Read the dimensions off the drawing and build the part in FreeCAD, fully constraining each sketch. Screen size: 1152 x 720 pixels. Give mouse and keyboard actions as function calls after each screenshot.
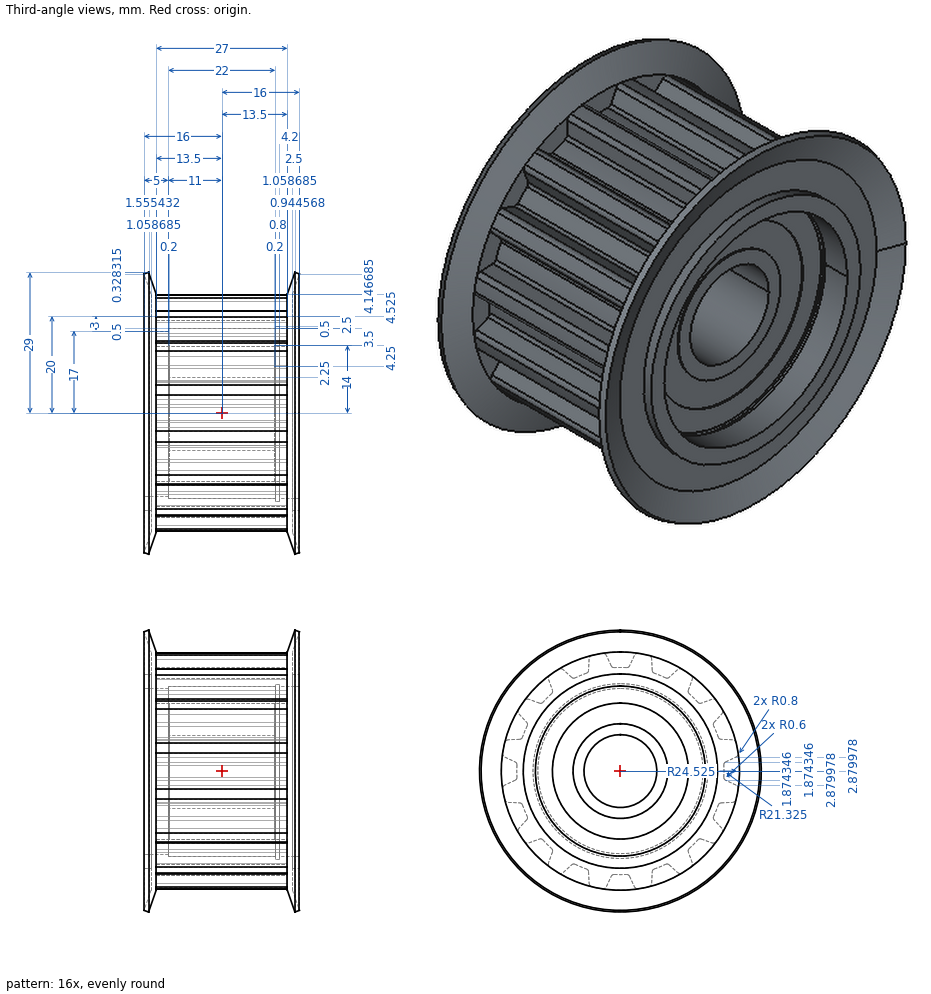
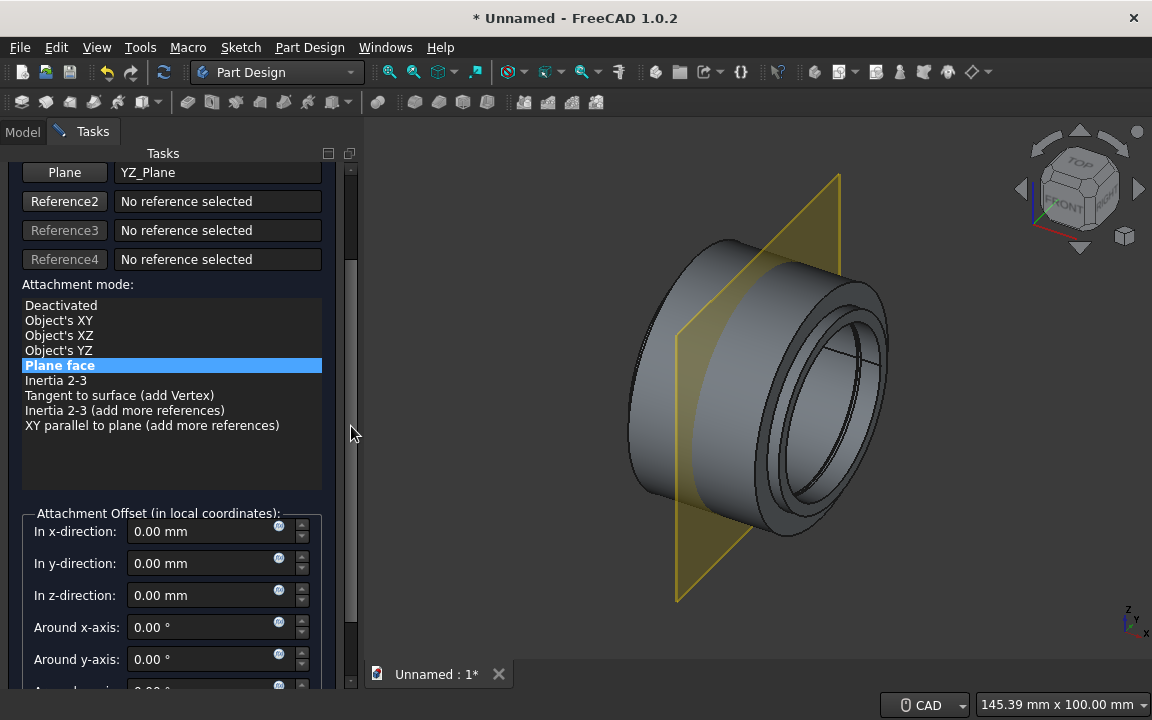
triple_click(210, 595)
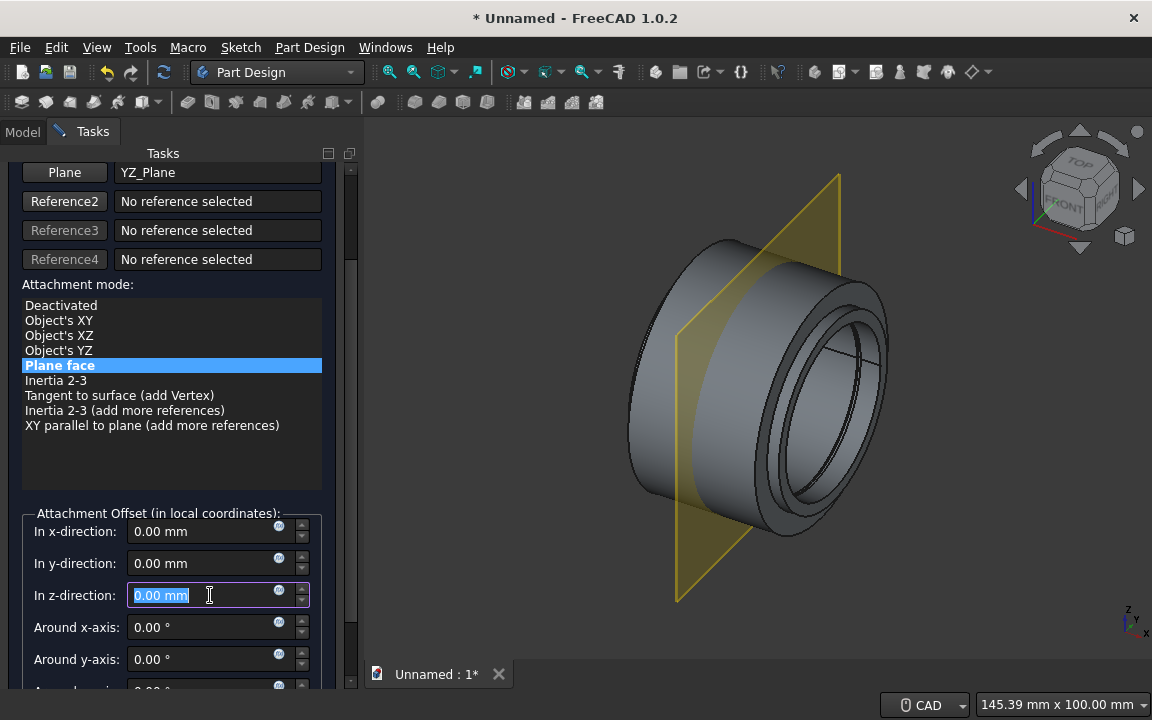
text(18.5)
key(Tab)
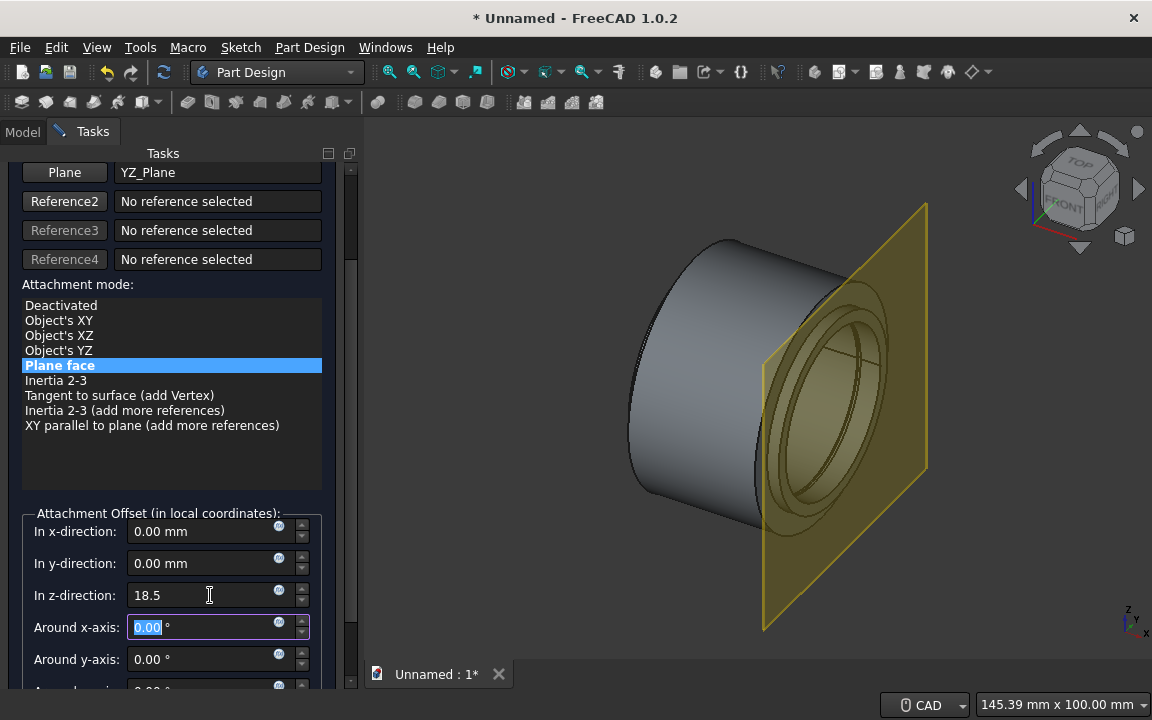
scroll(351, 426, up, 3)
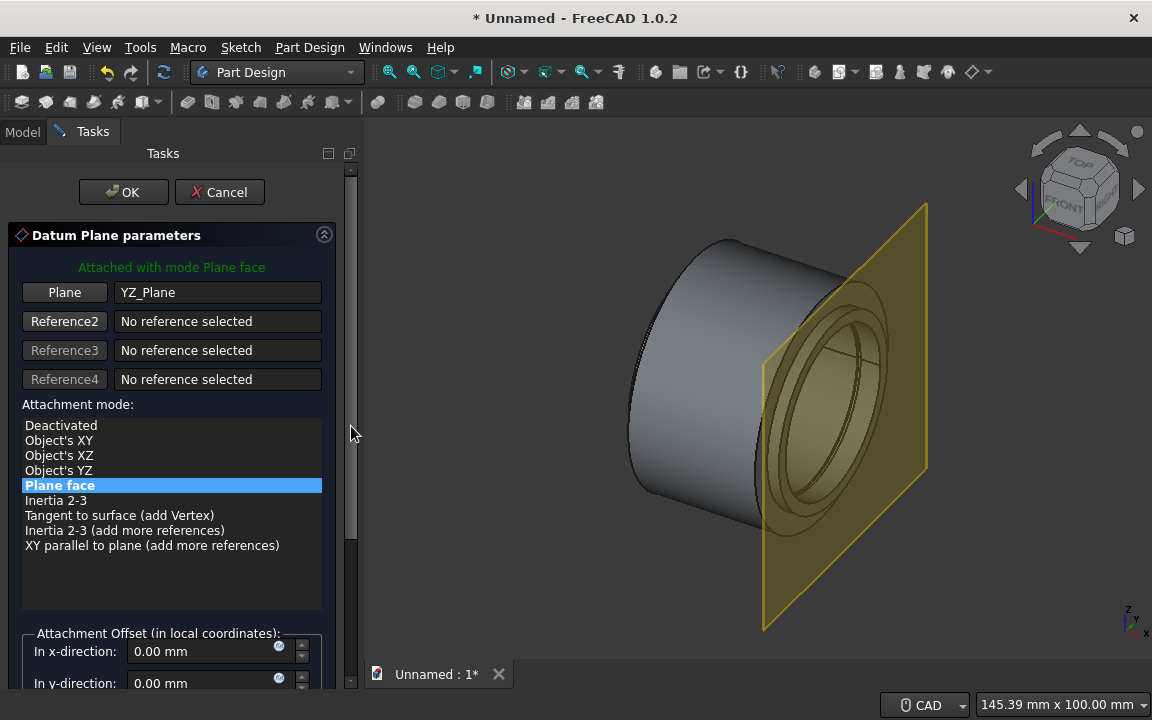
click(124, 192)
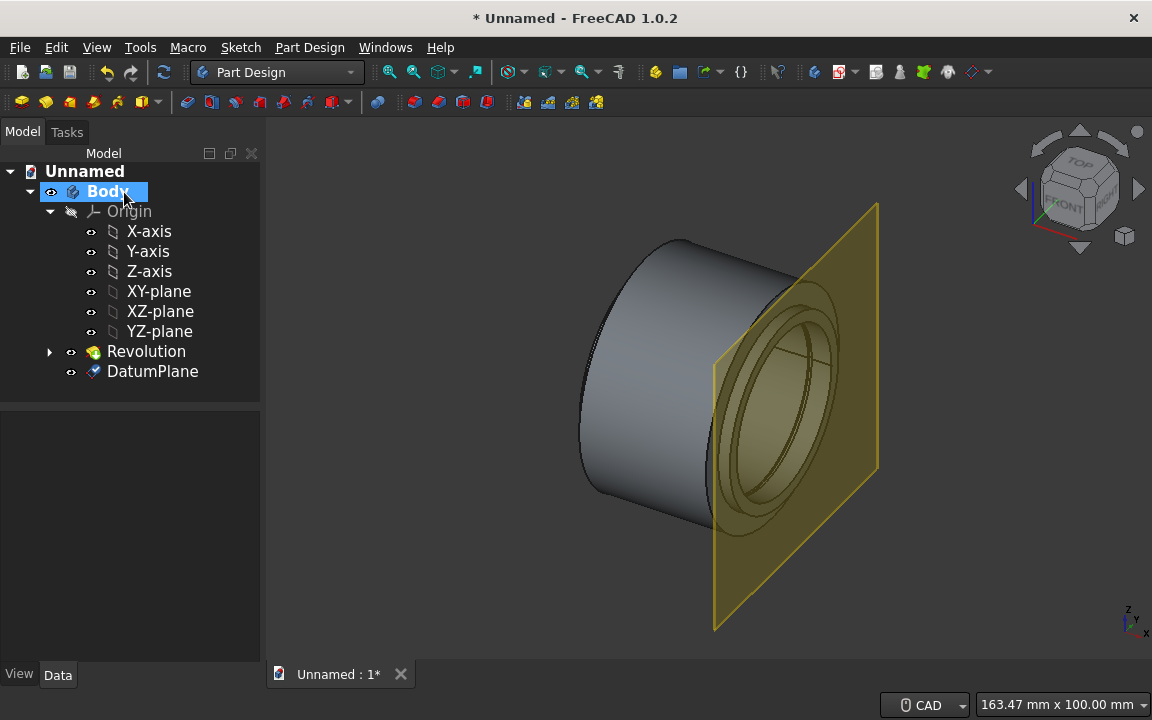
click(116, 372)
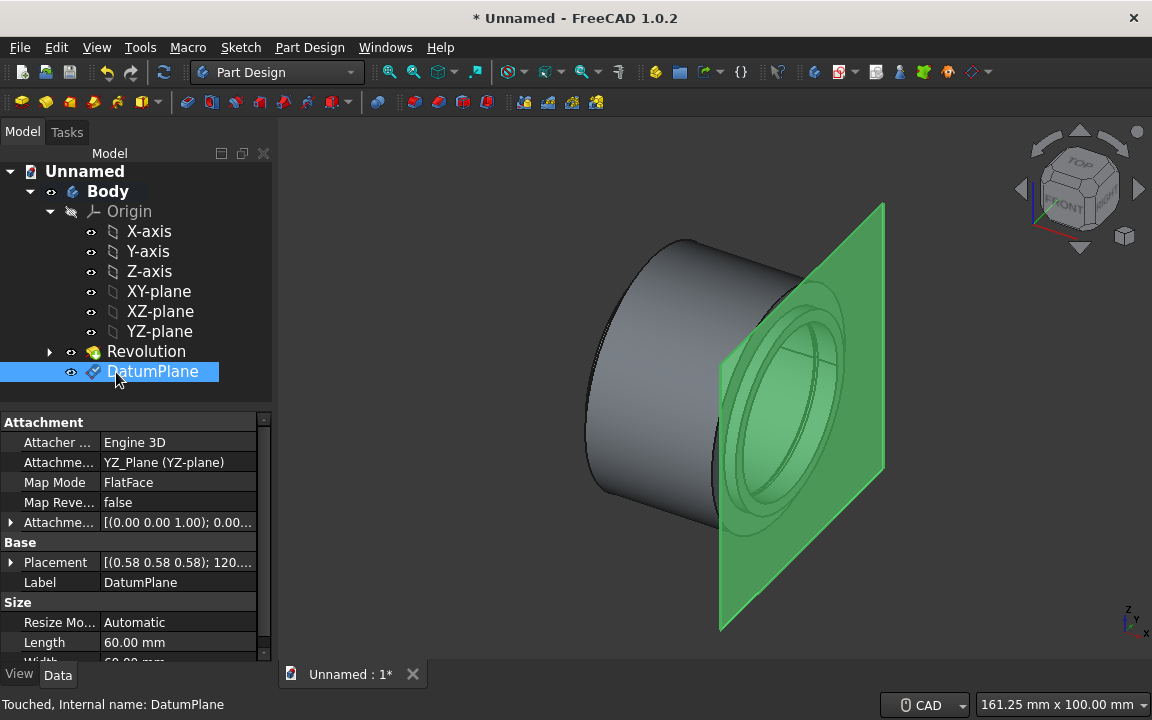
click(840, 72)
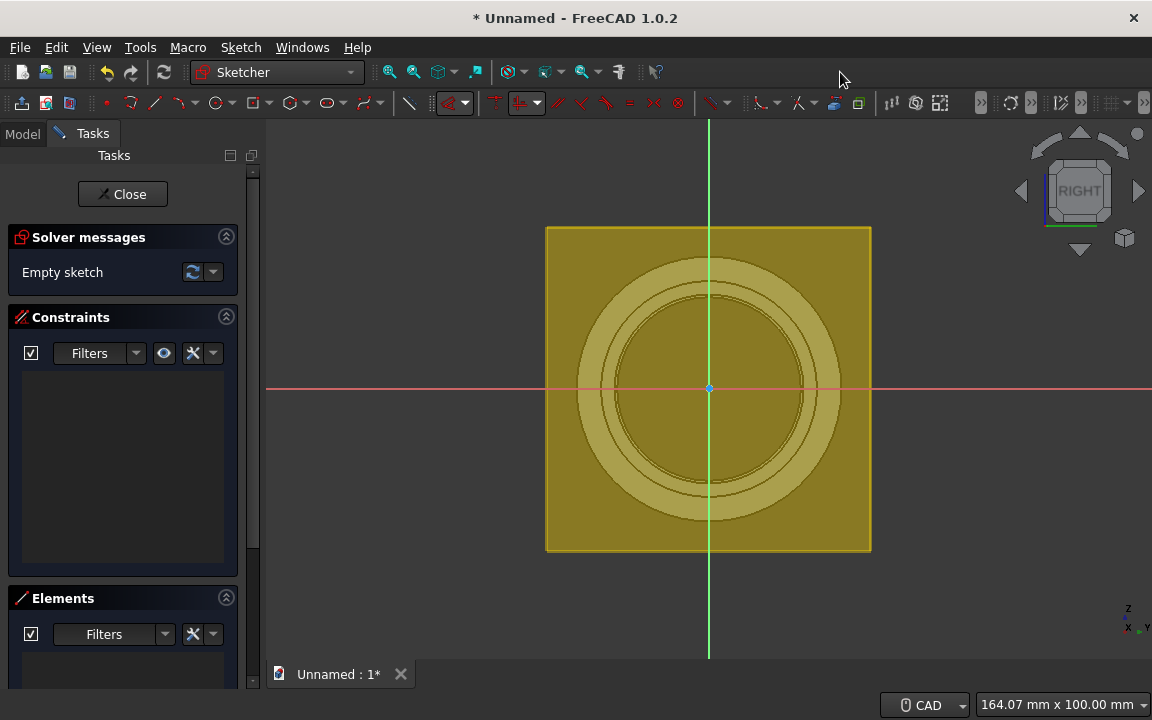
scroll(857, 389, up, 11)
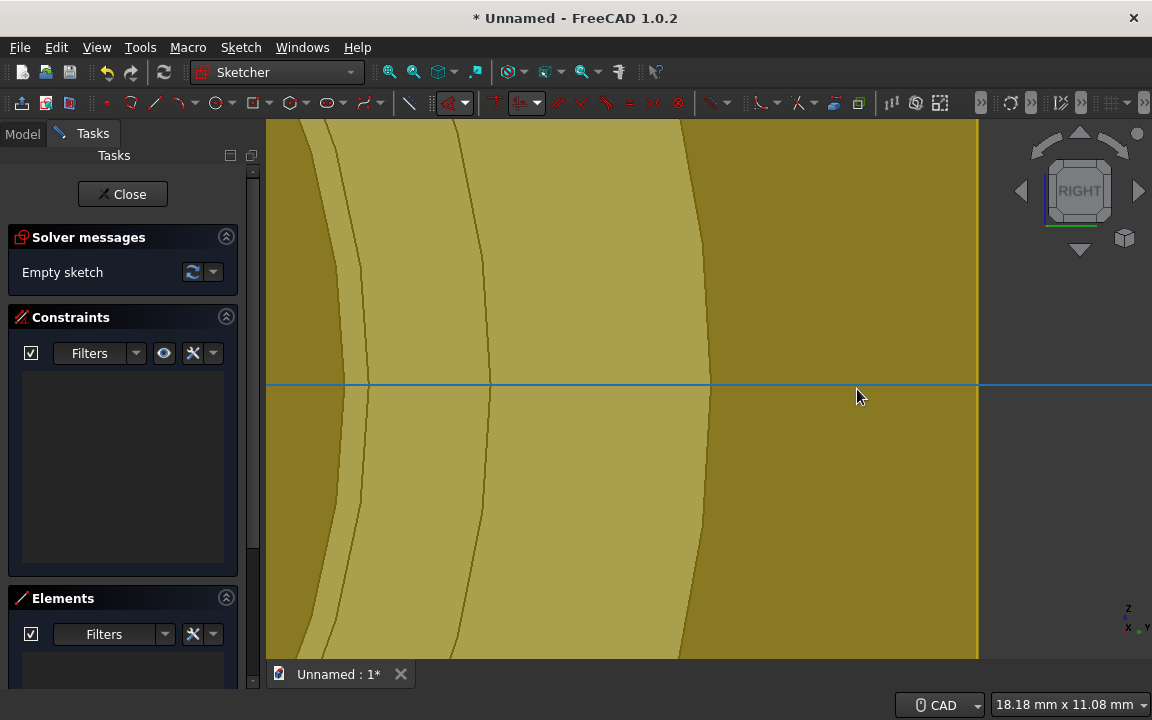
click(156, 104)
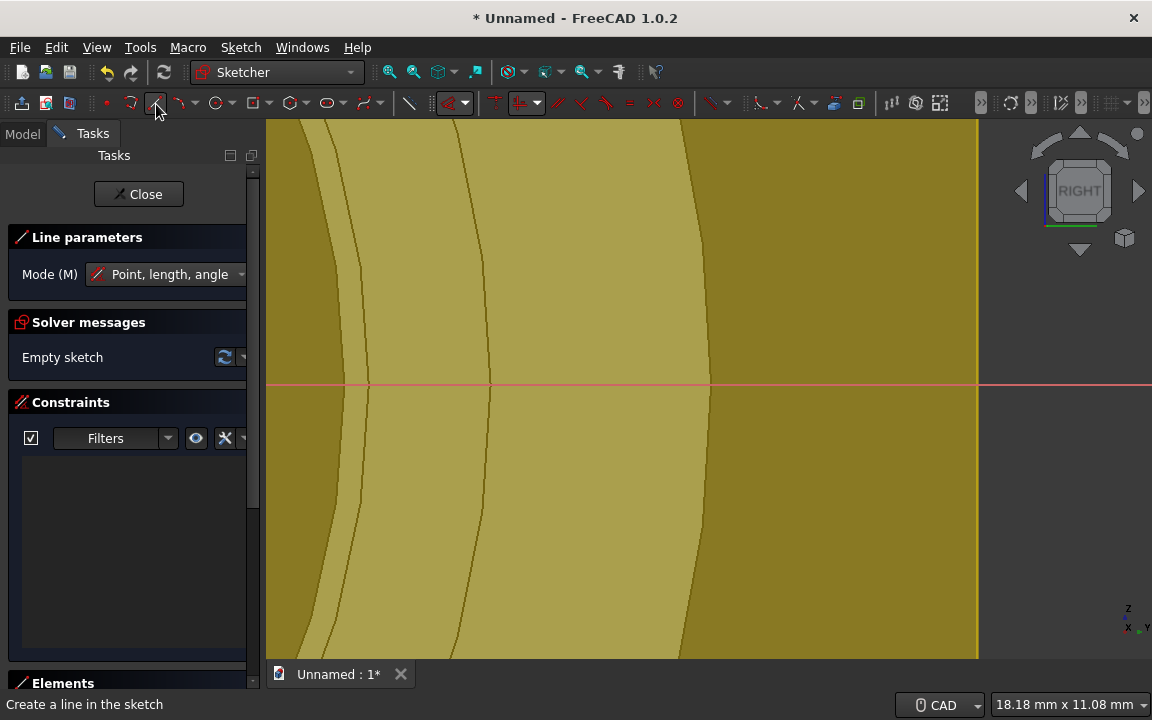
click(675, 525)
click(570, 476)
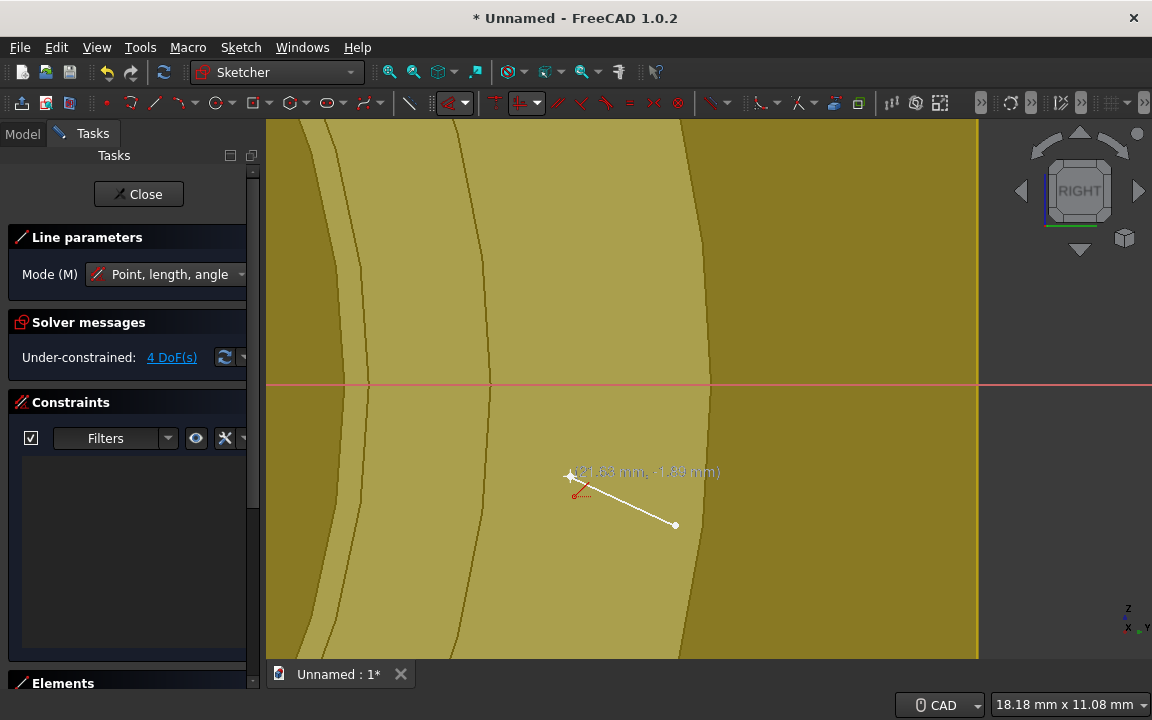
click(570, 294)
click(675, 245)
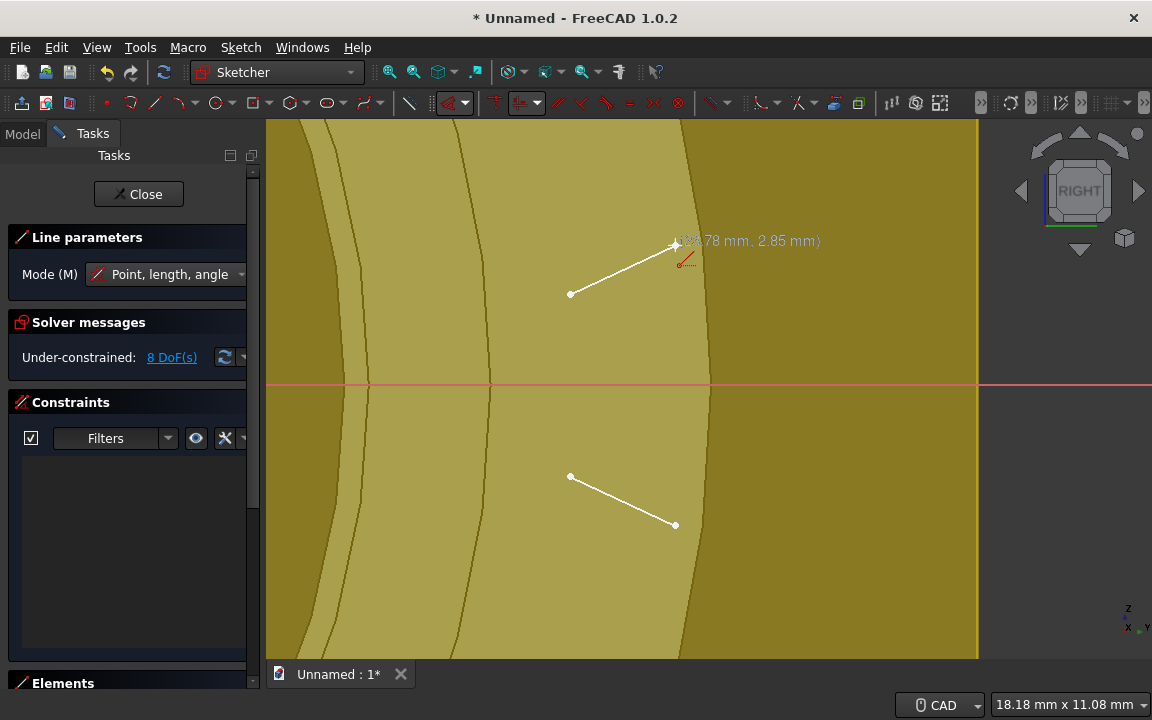
click(180, 104)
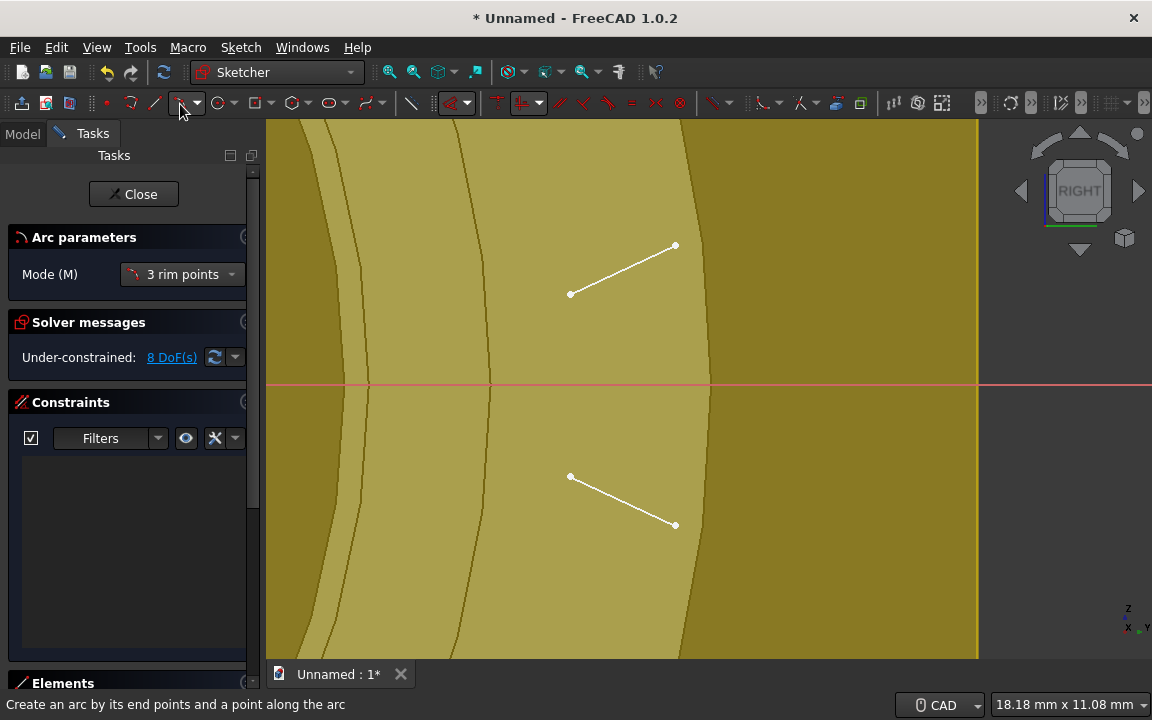
click(570, 477)
click(553, 448)